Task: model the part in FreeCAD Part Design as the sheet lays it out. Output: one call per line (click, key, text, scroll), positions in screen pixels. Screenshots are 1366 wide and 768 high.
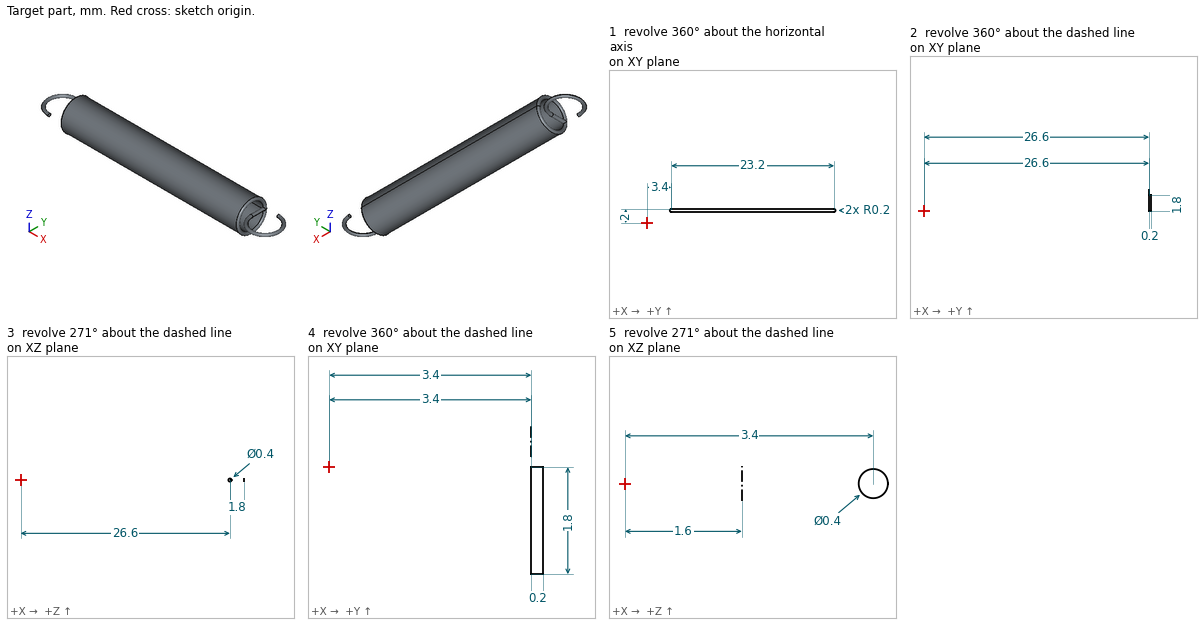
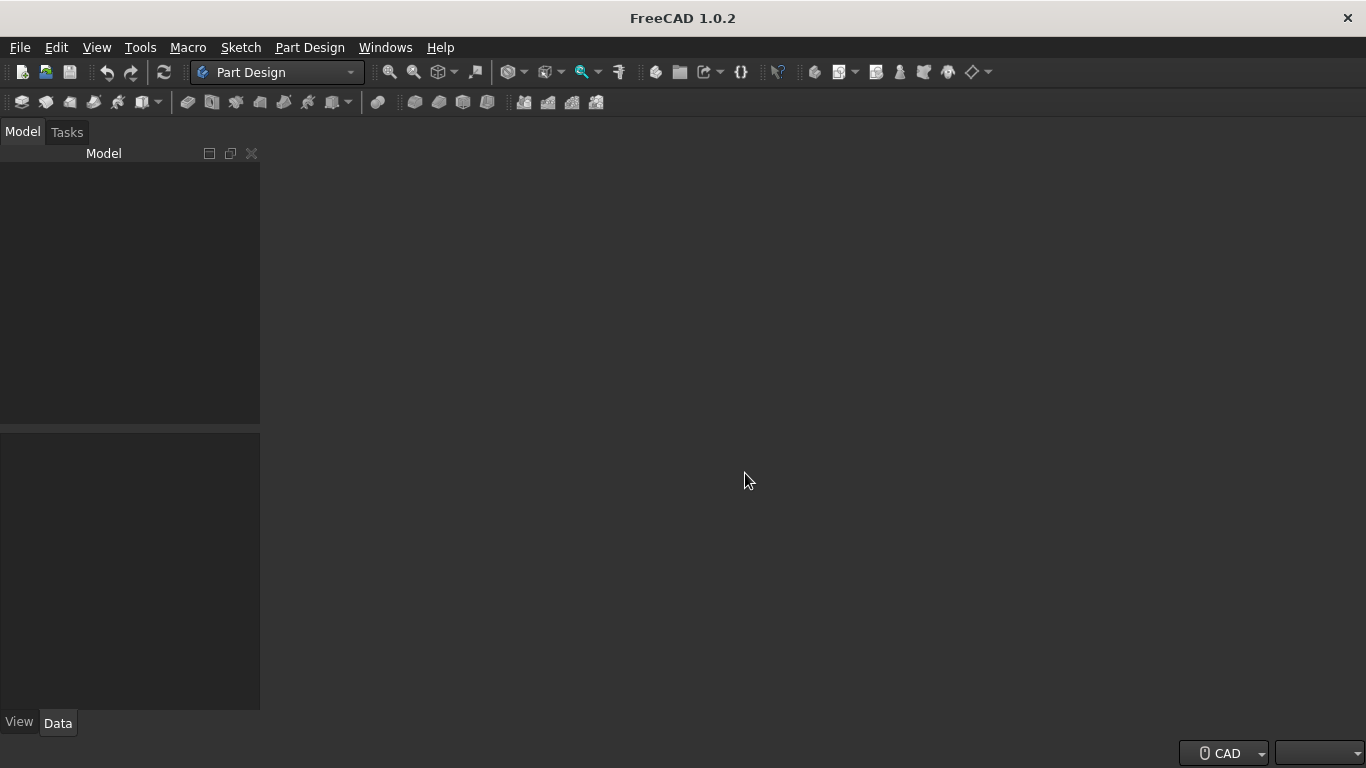
click(22, 72)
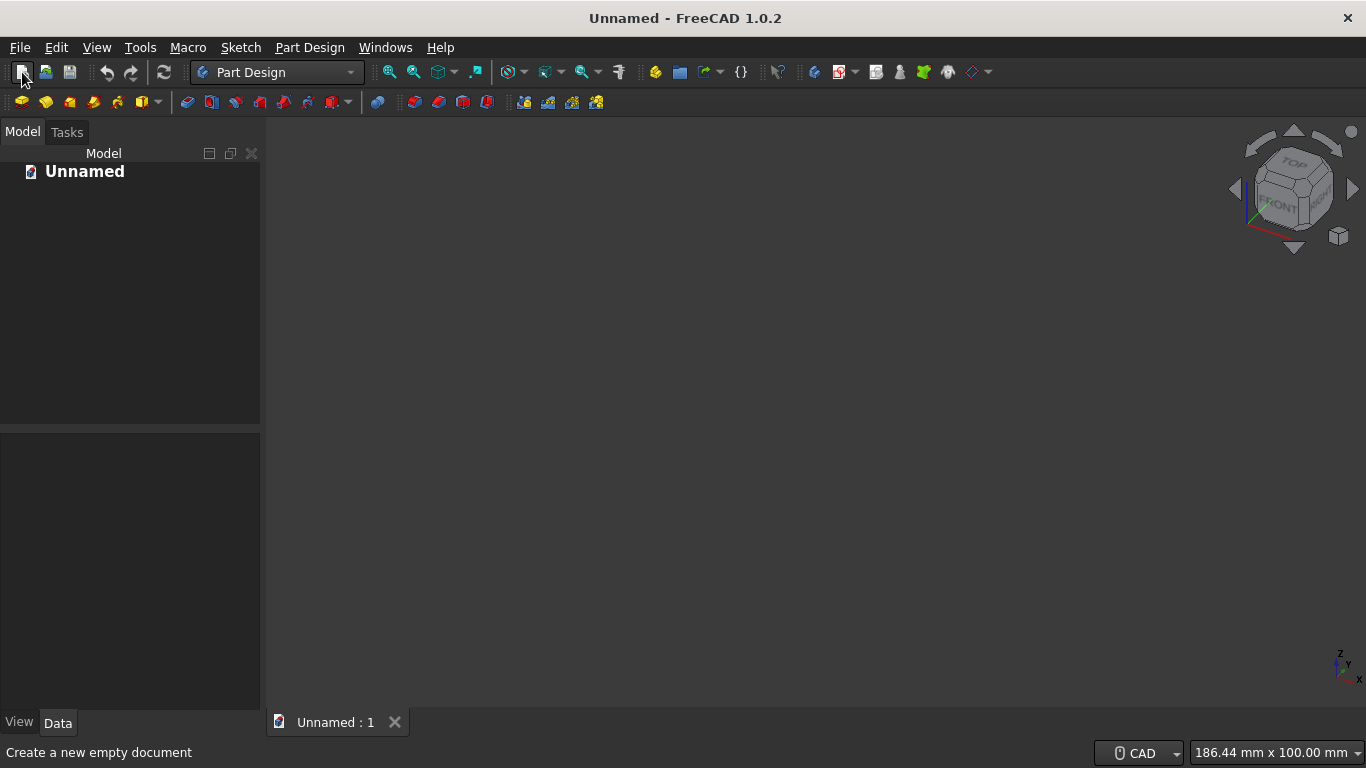
click(840, 72)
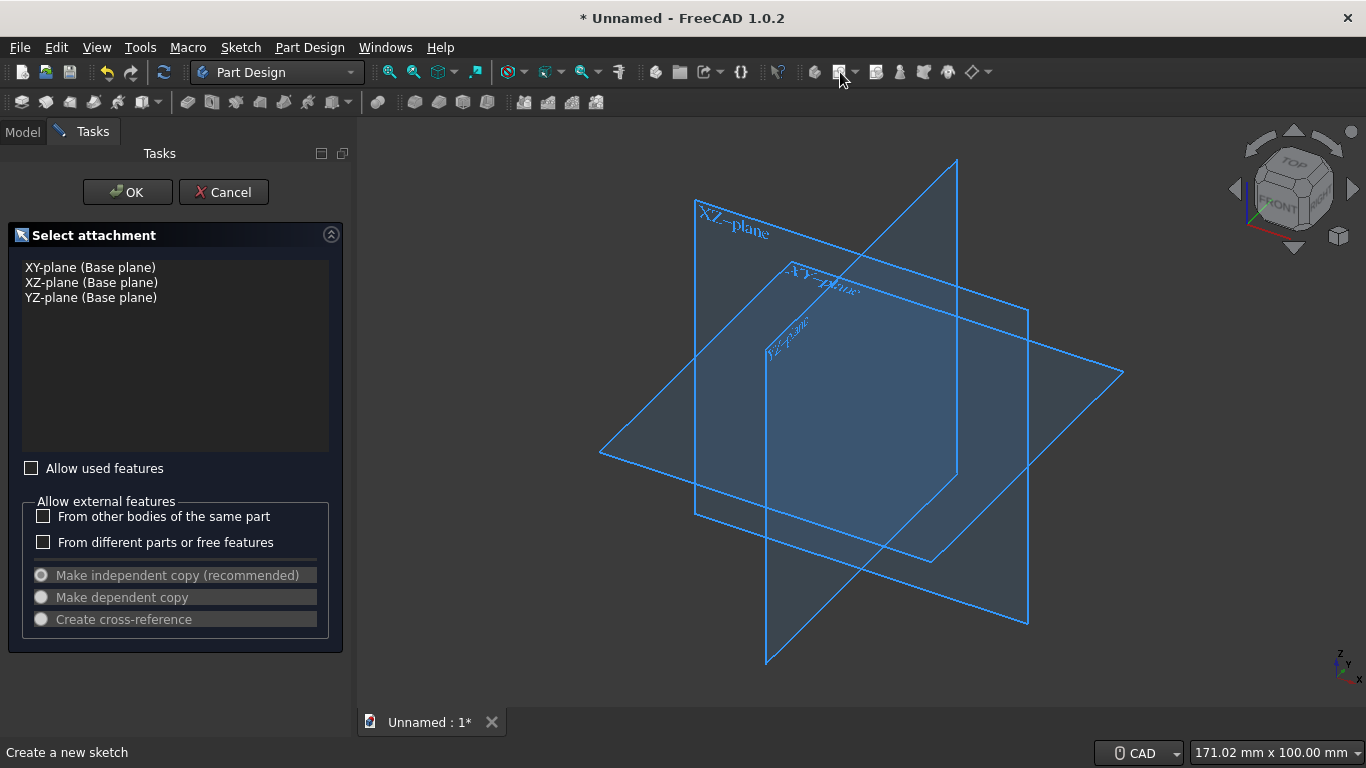
click(82, 268)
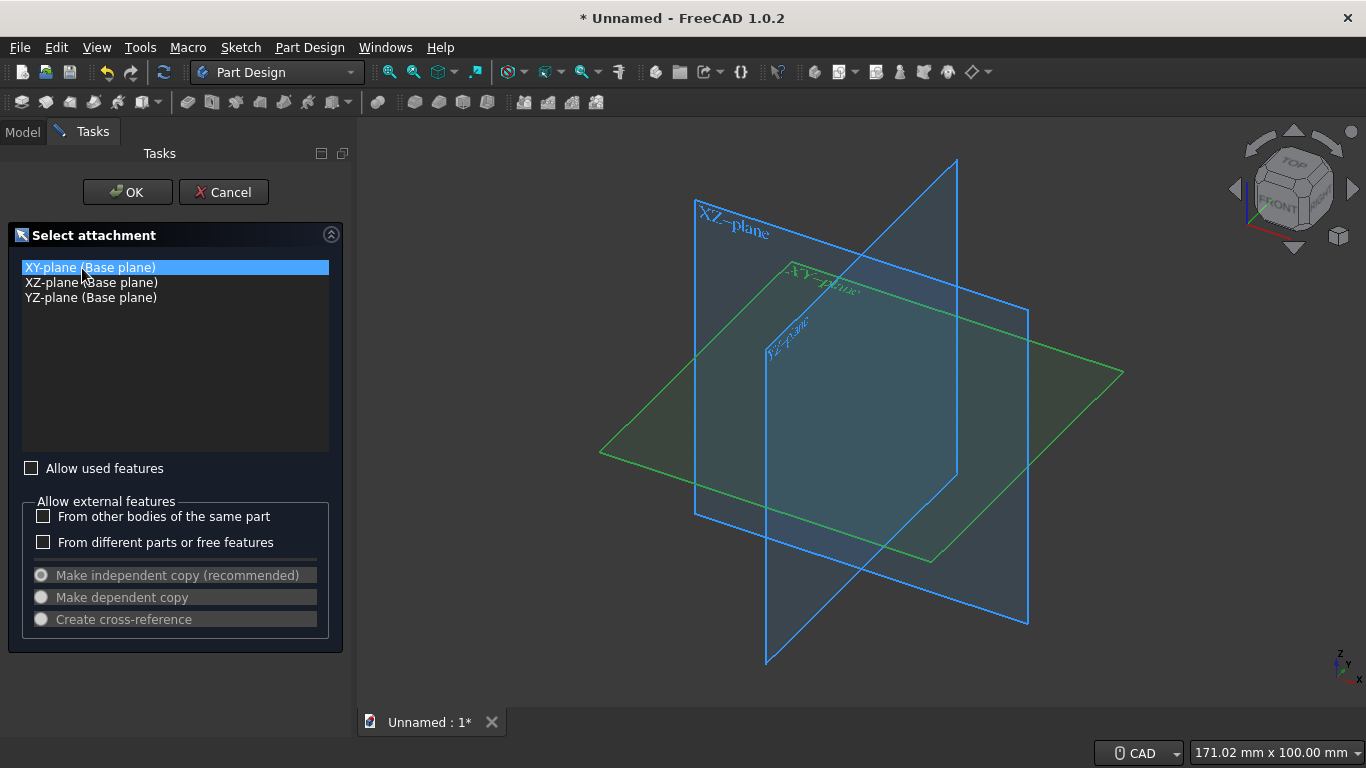
click(128, 192)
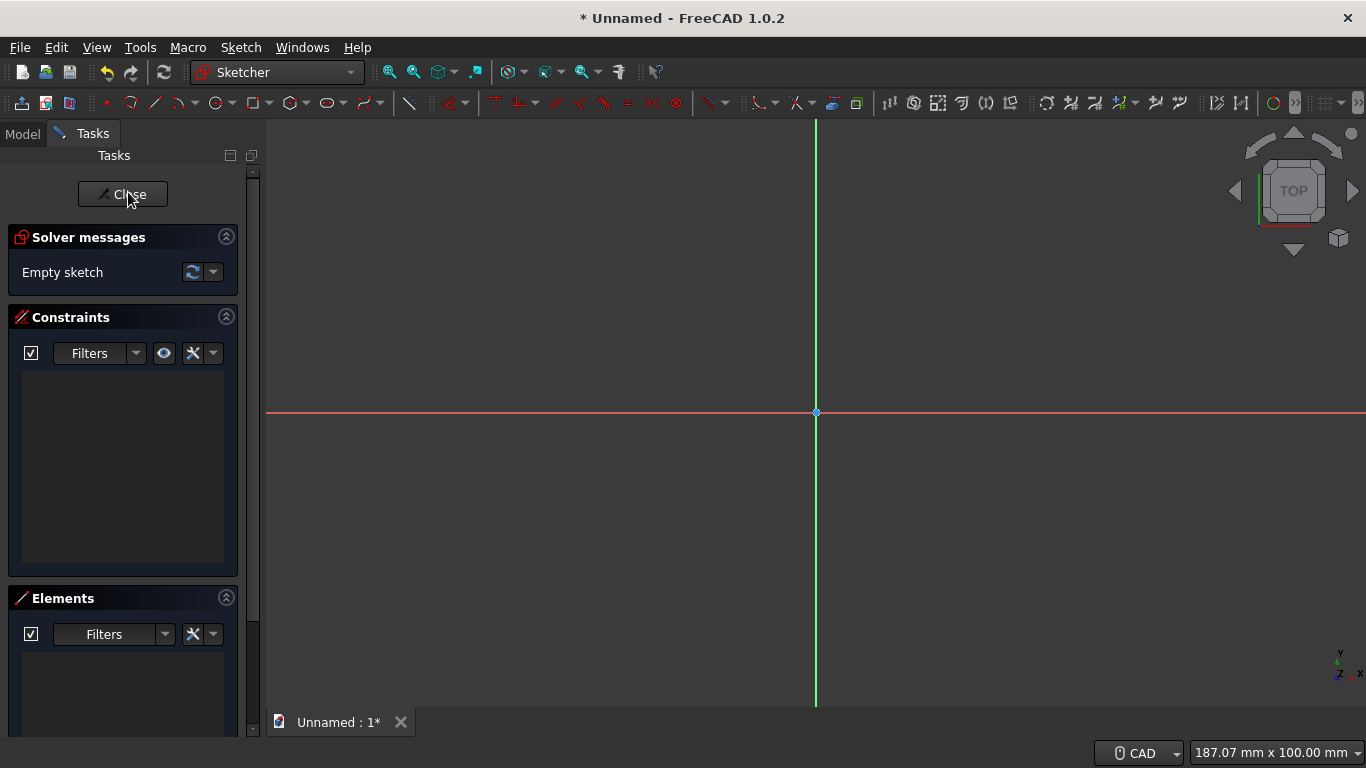
scroll(943, 405, up, 7)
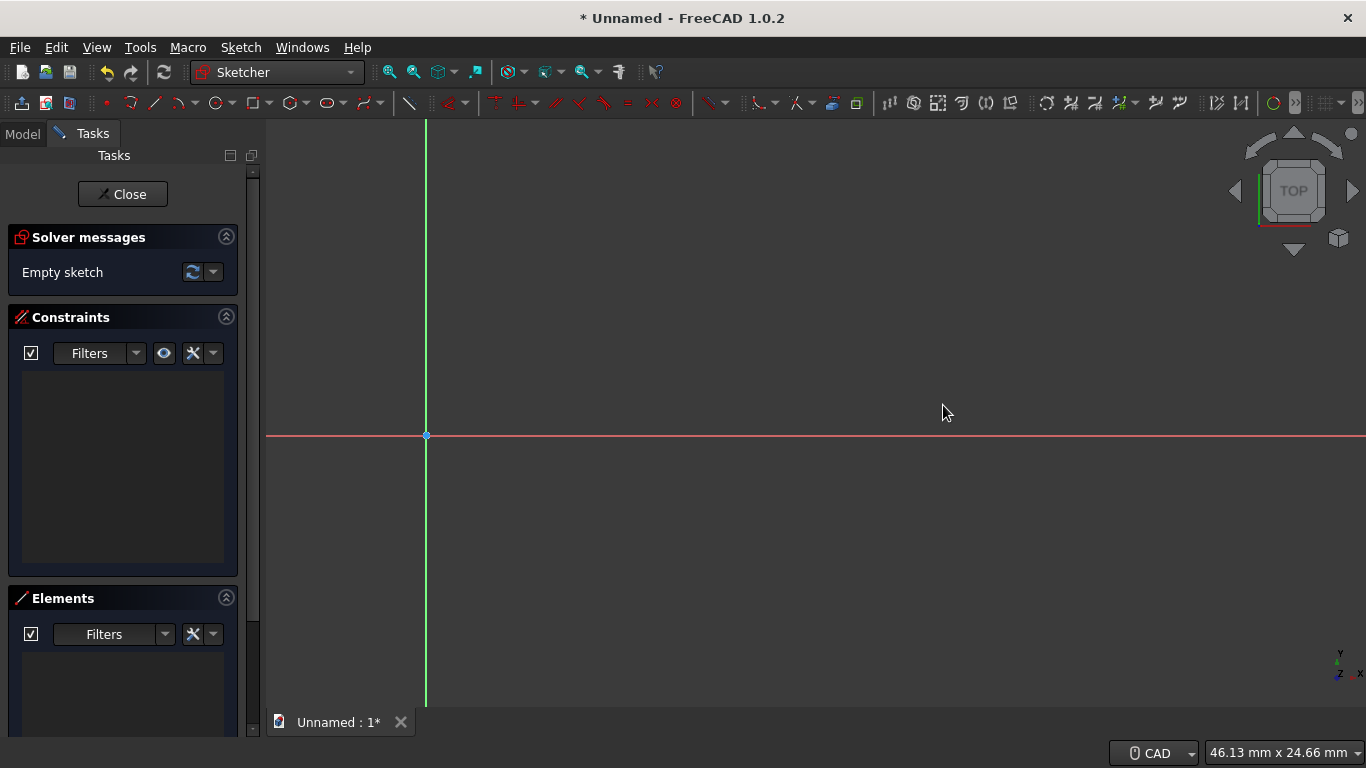
click(328, 104)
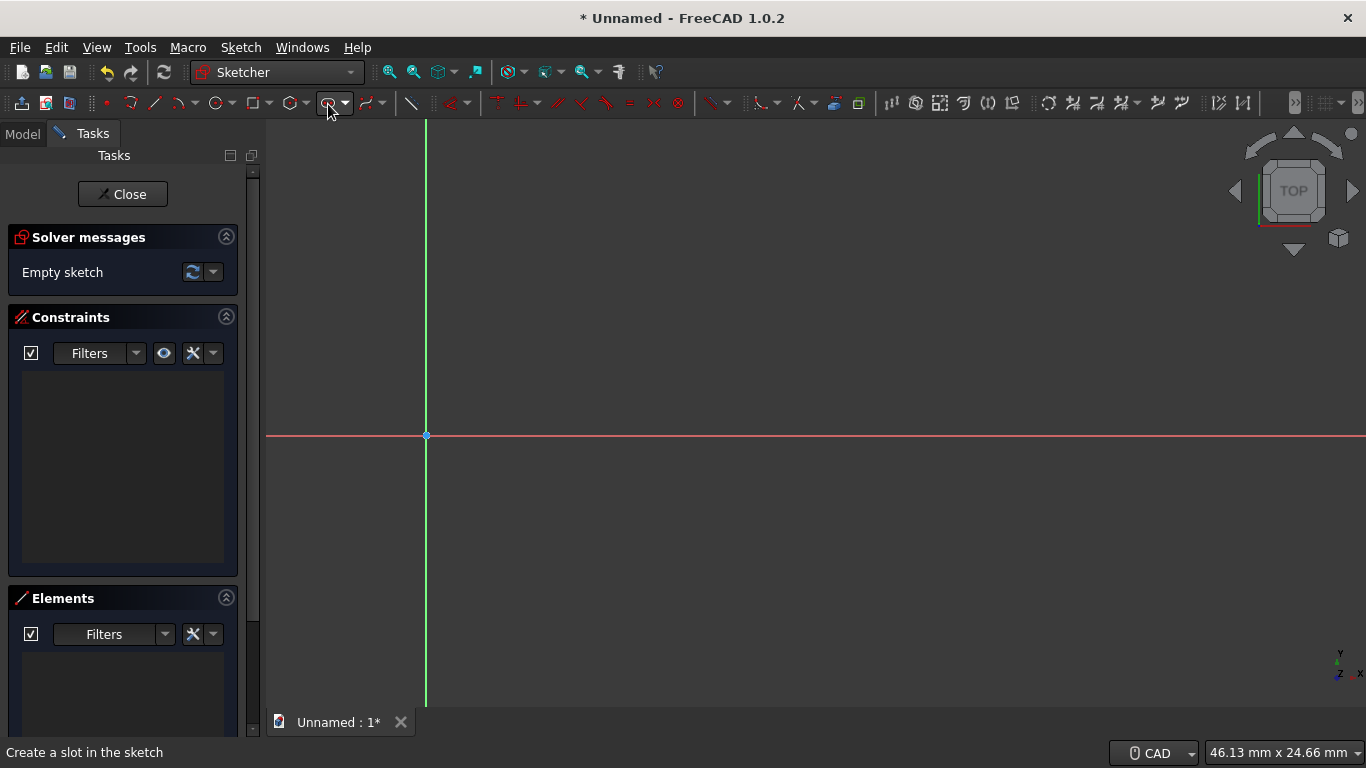
scroll(507, 393, up, 8)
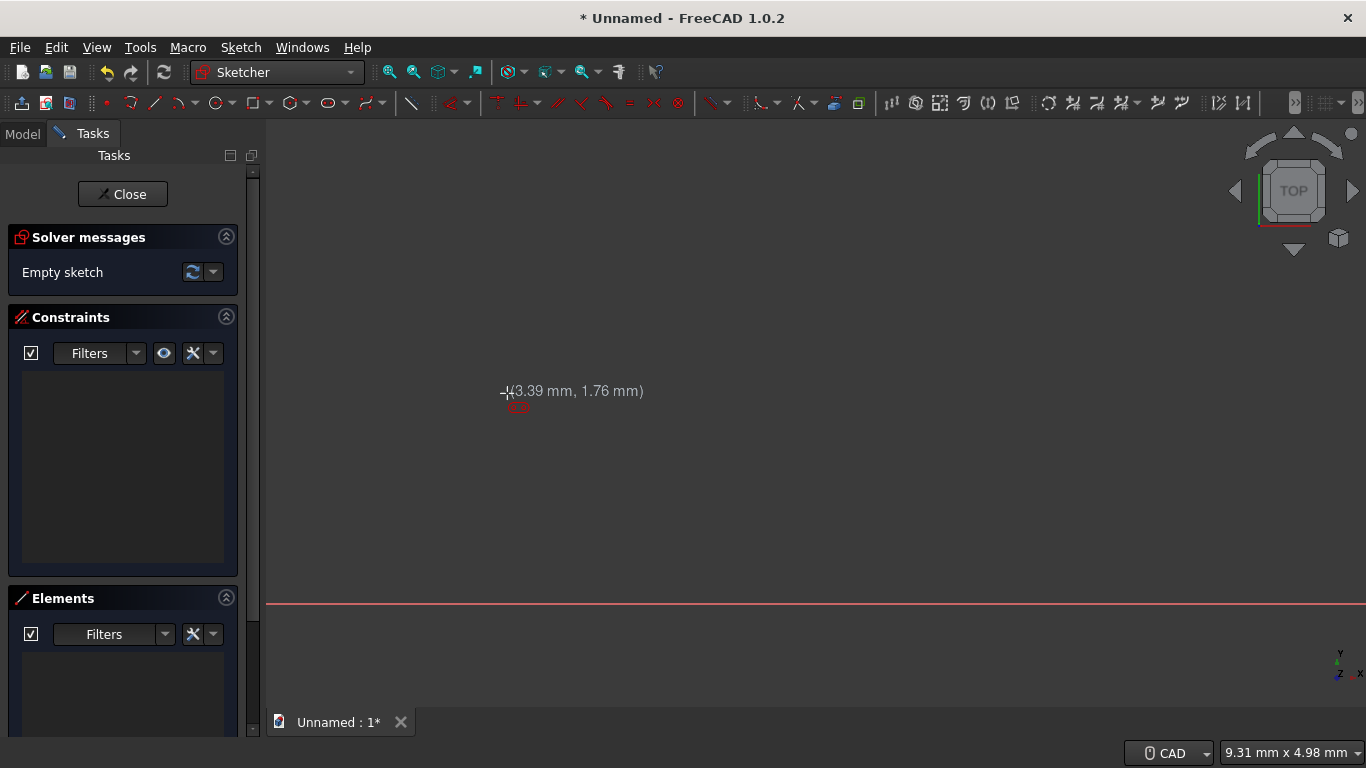
scroll(510, 395, down, 8)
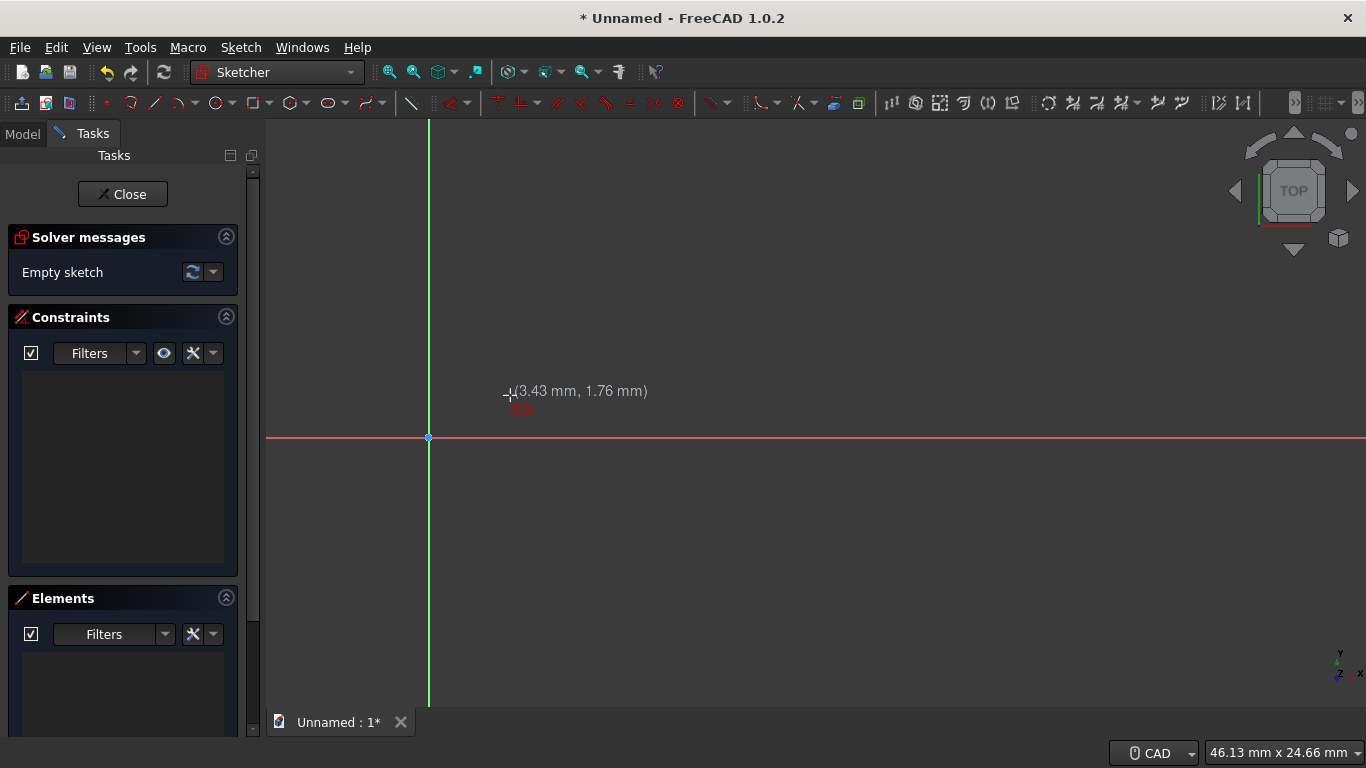
click(510, 395)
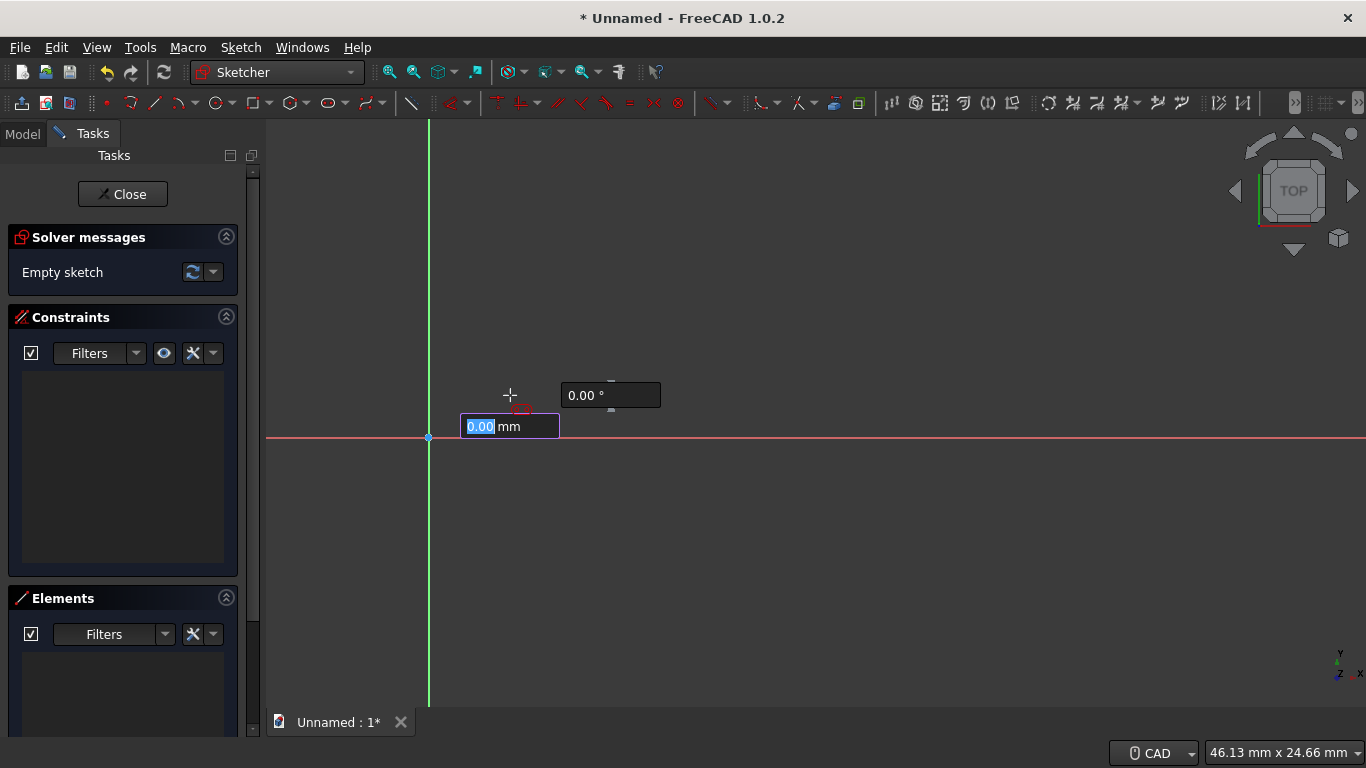
click(1063, 395)